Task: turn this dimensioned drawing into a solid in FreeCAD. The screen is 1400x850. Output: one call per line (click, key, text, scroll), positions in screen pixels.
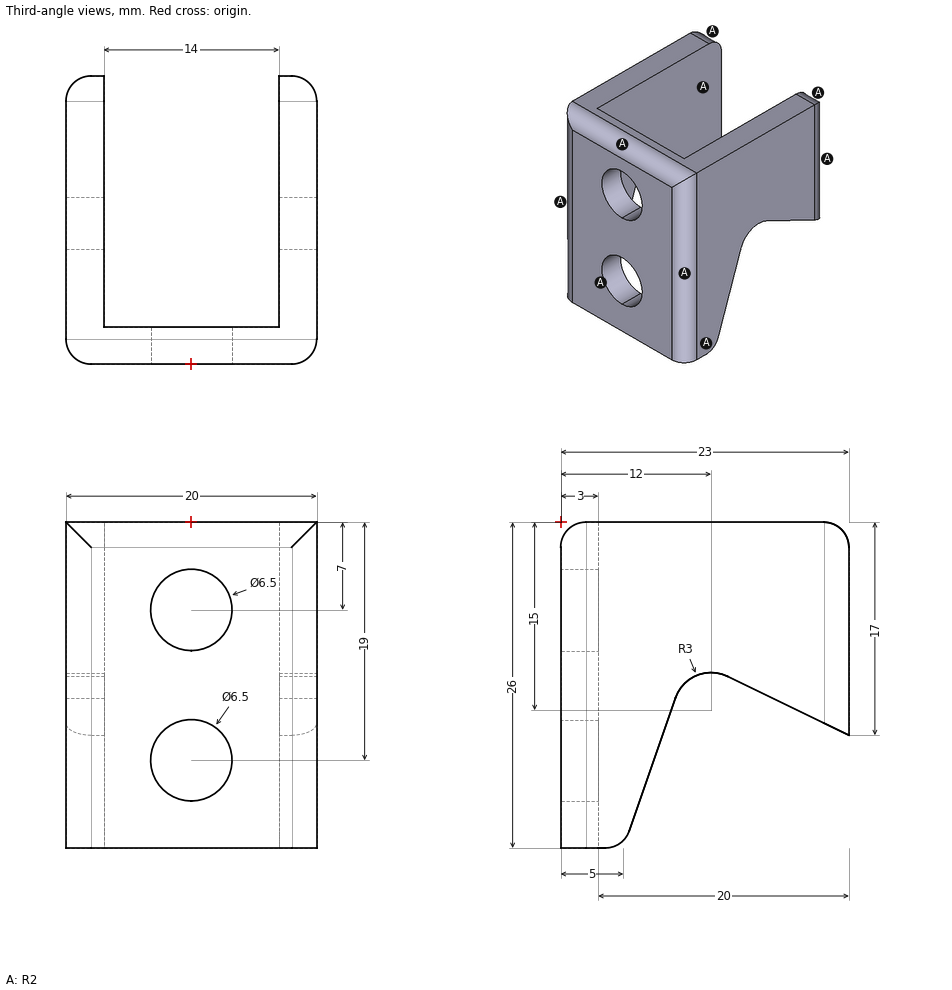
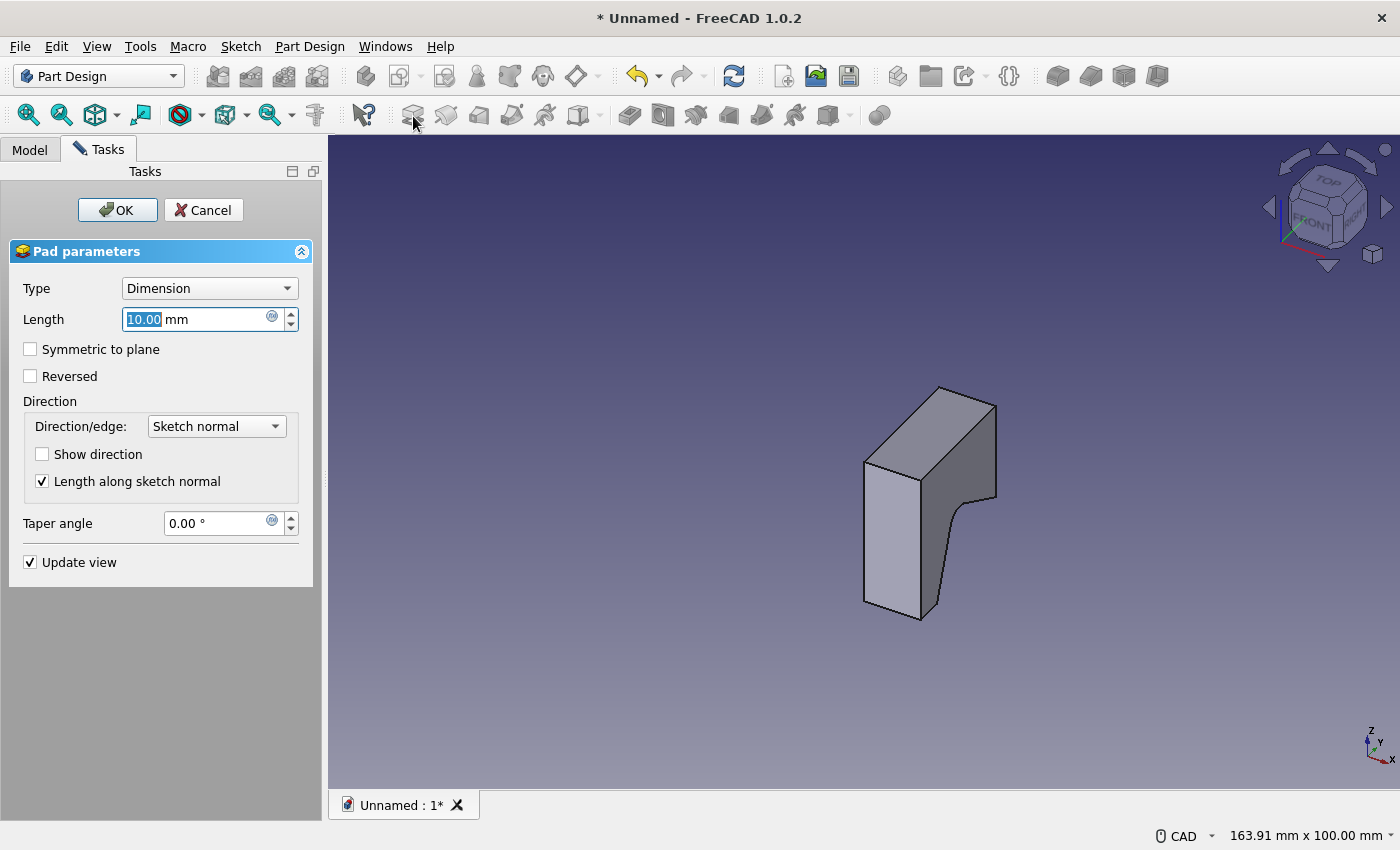
text(20)
key(Tab)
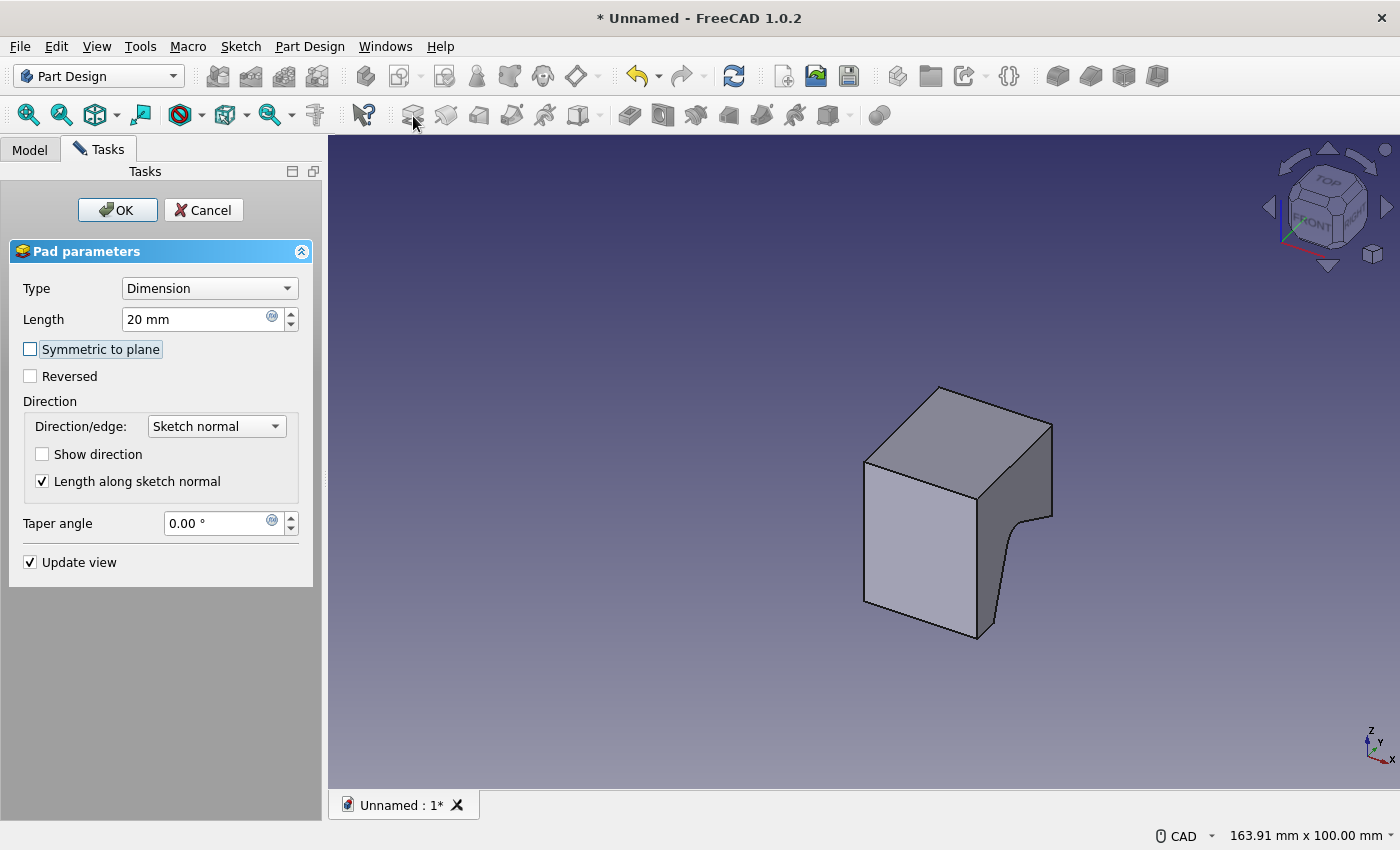
click(31, 349)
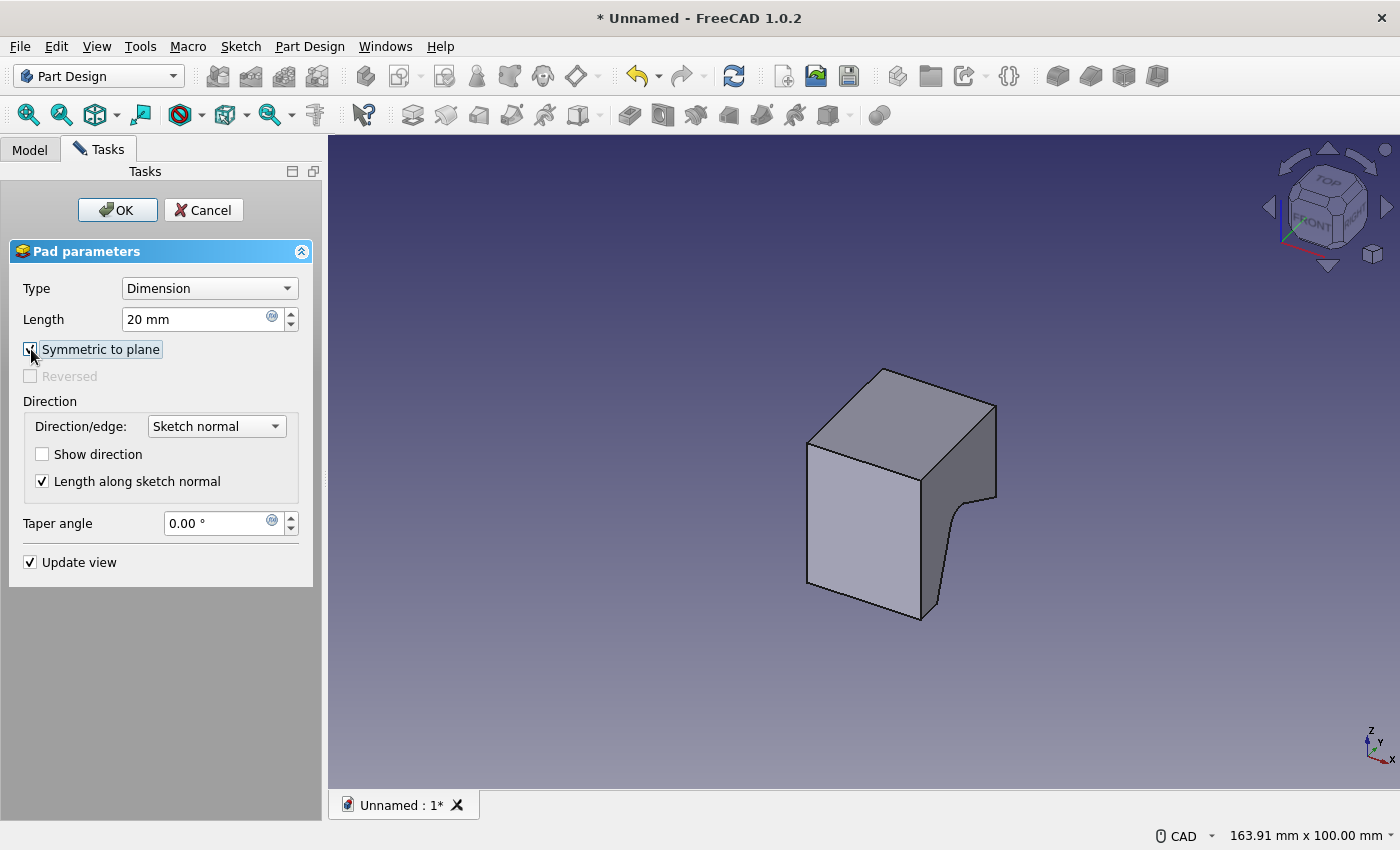
click(118, 210)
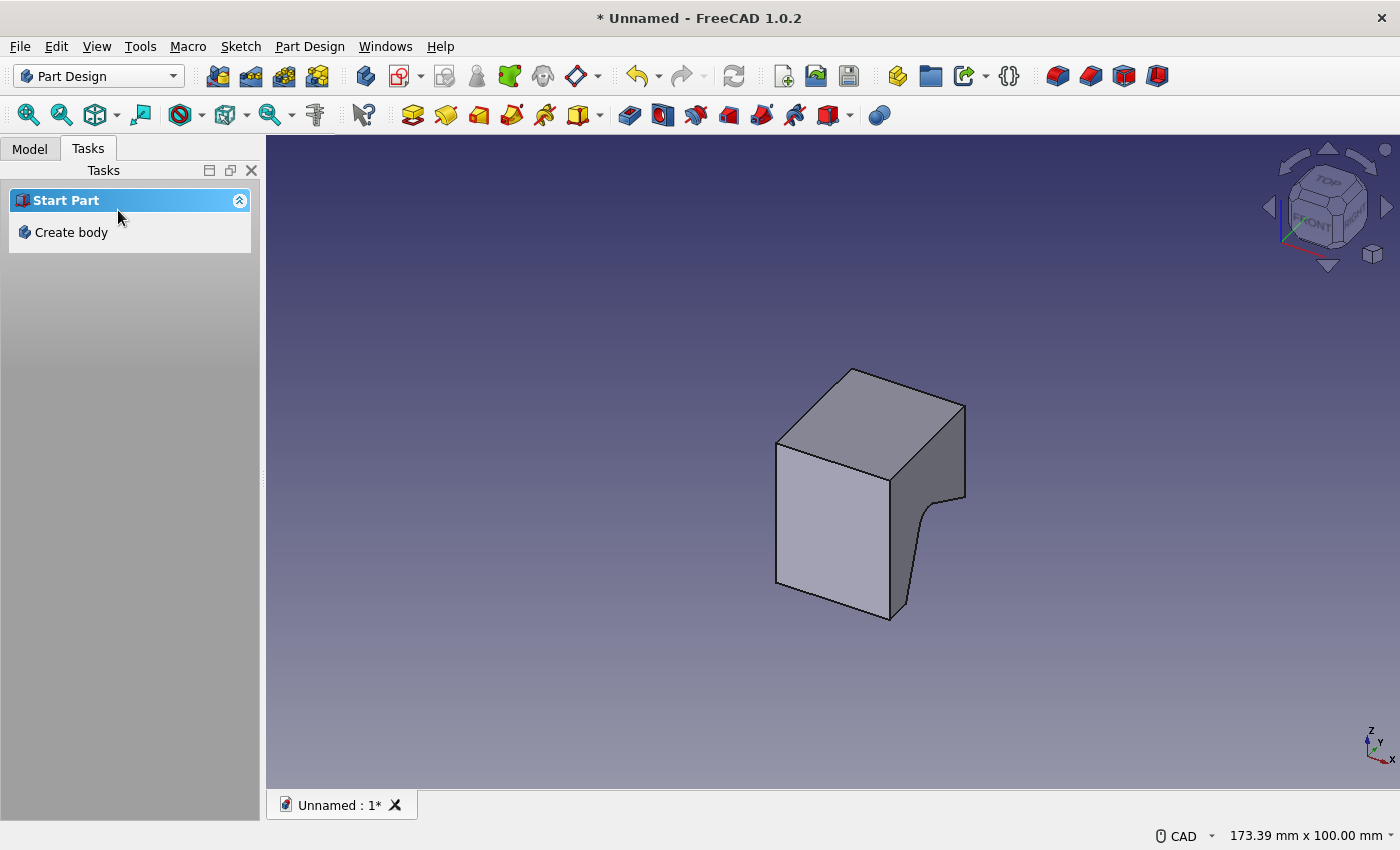
click(29, 116)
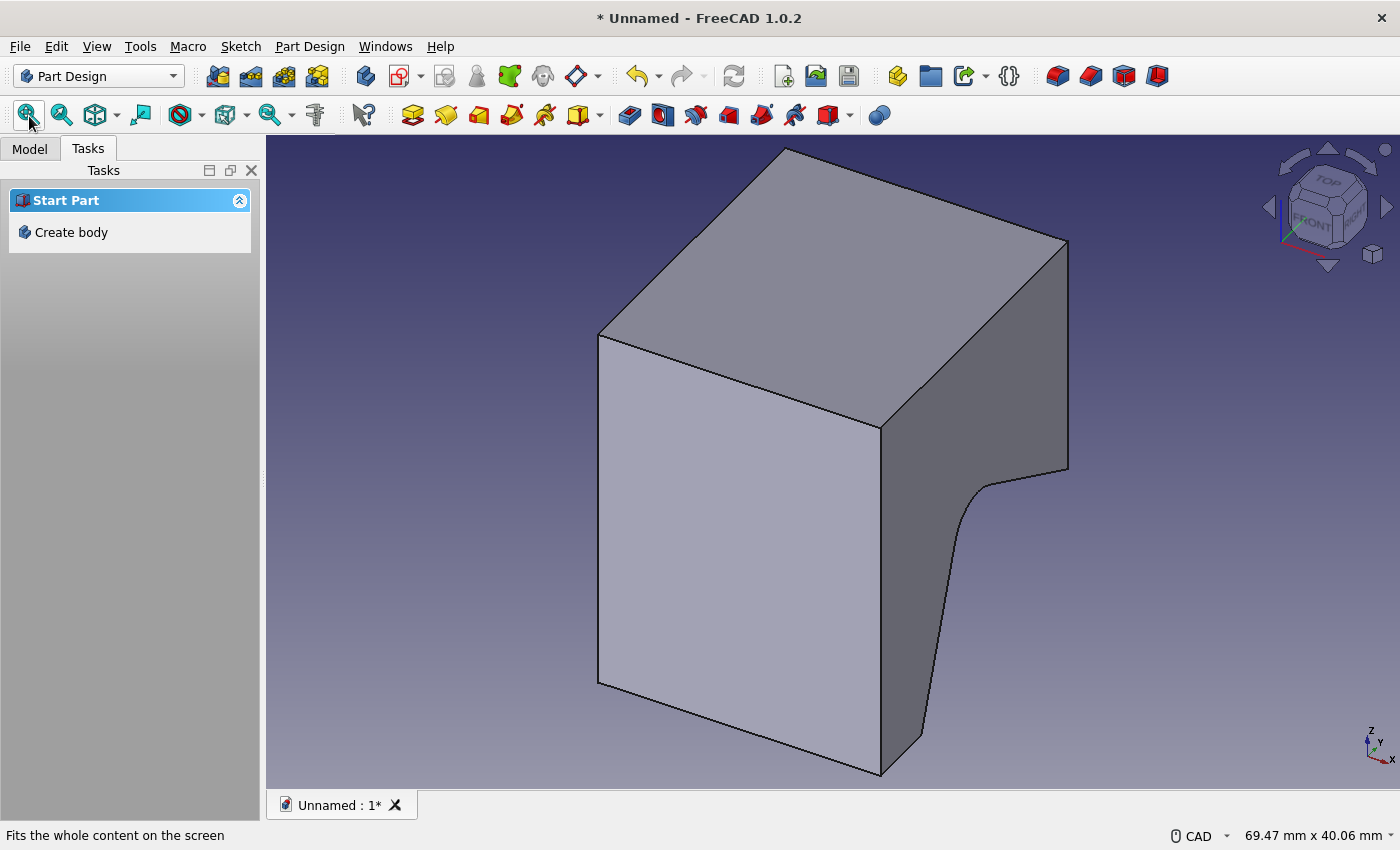
click(398, 76)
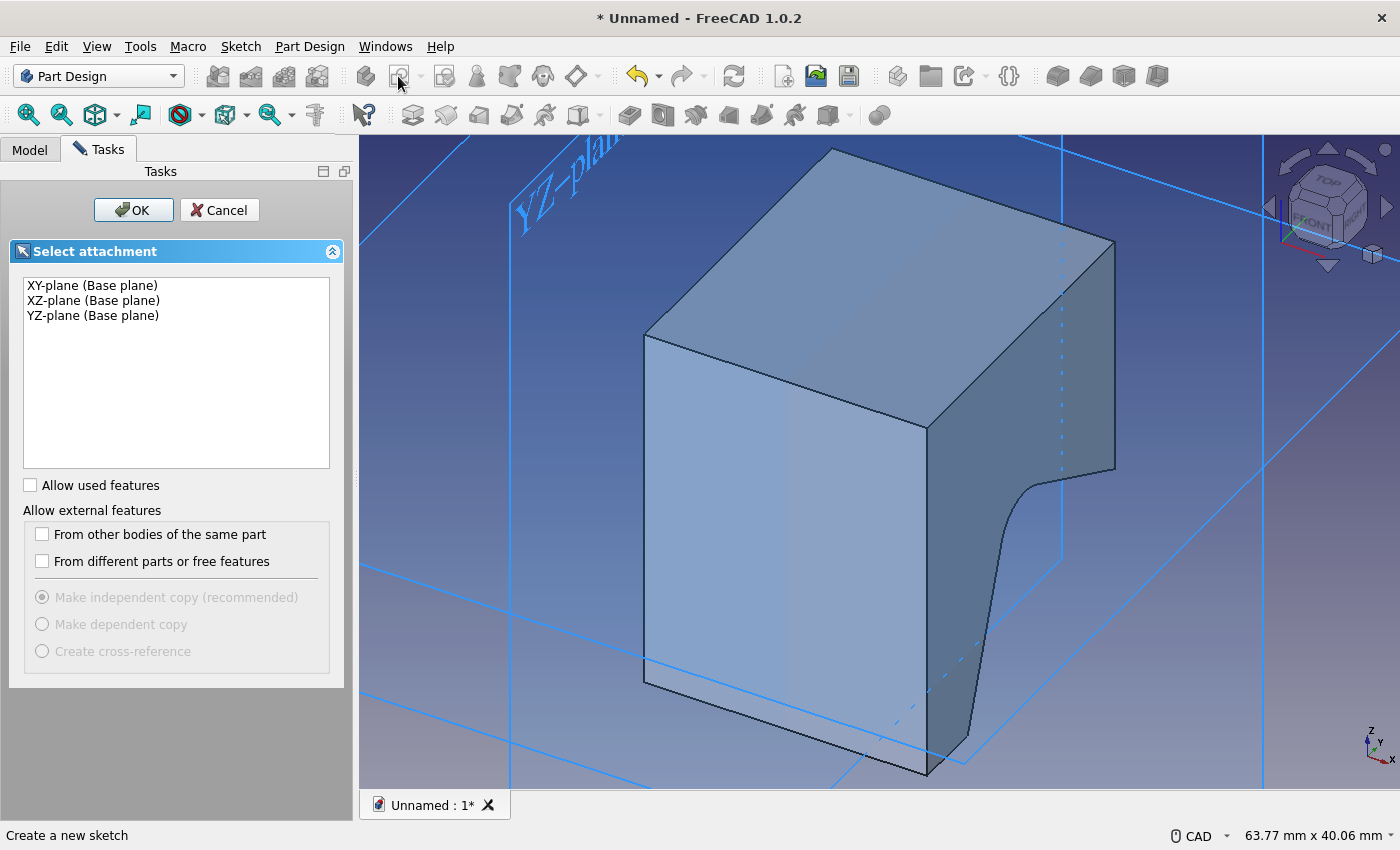
click(84, 316)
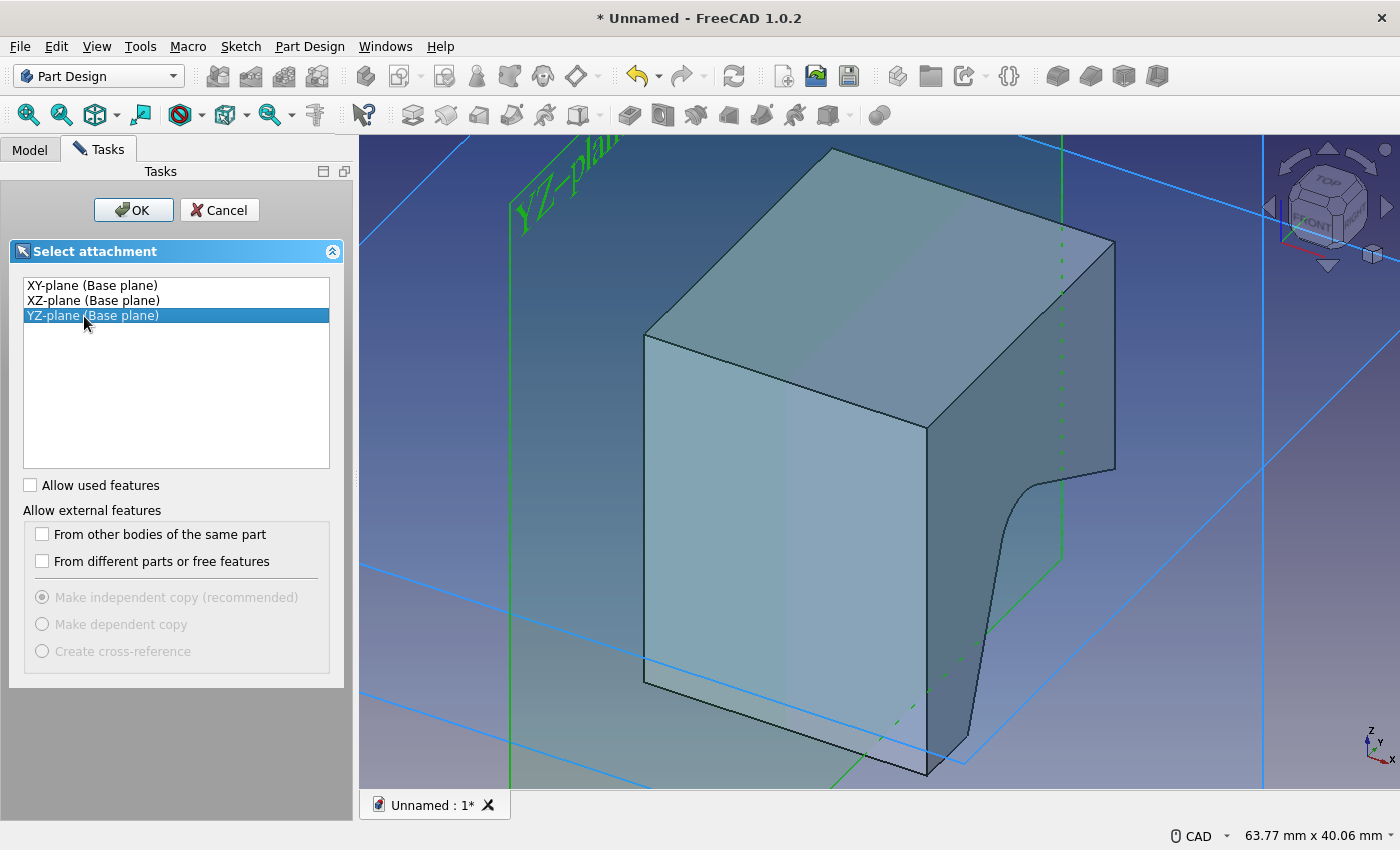
click(134, 210)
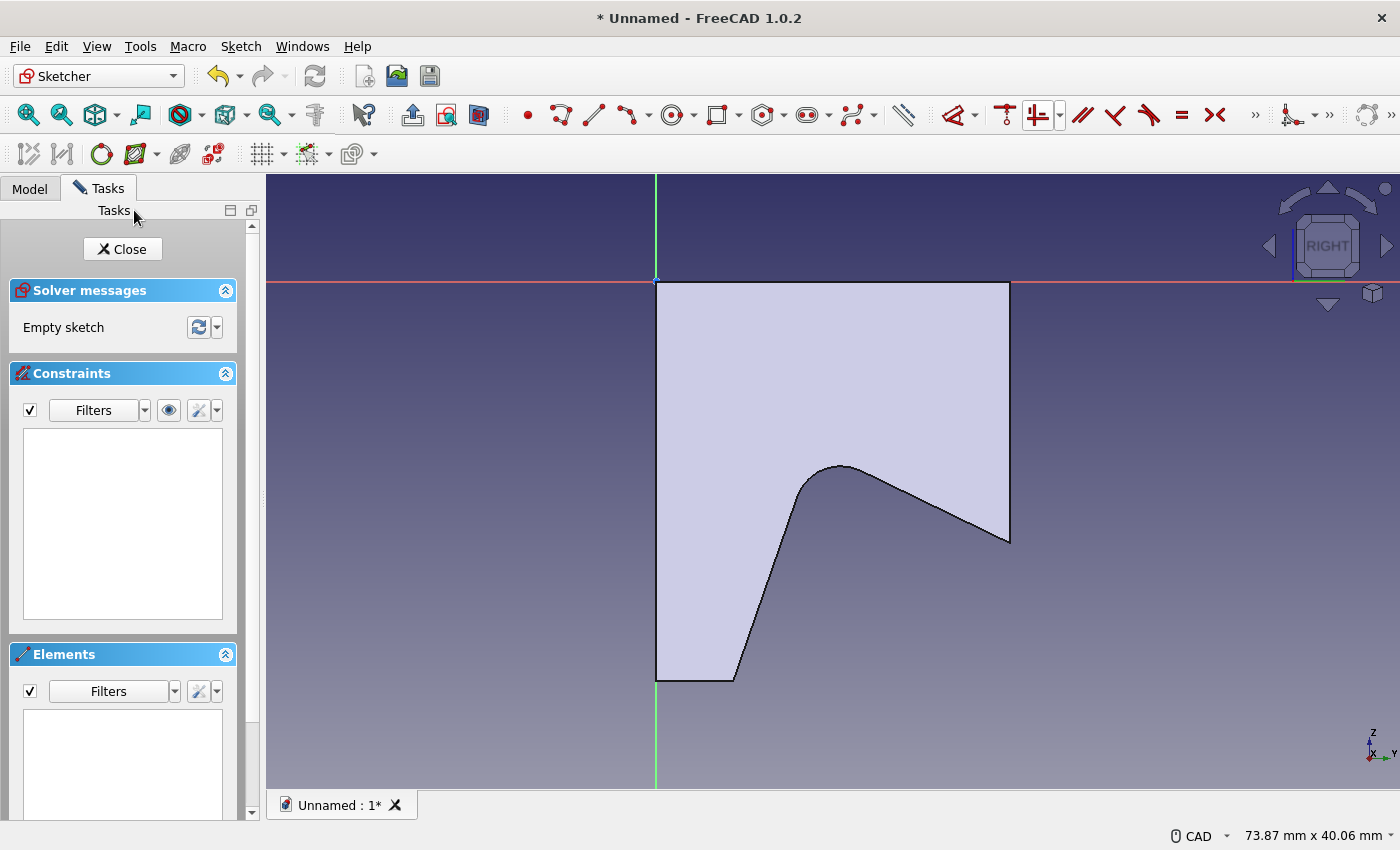
click(479, 116)